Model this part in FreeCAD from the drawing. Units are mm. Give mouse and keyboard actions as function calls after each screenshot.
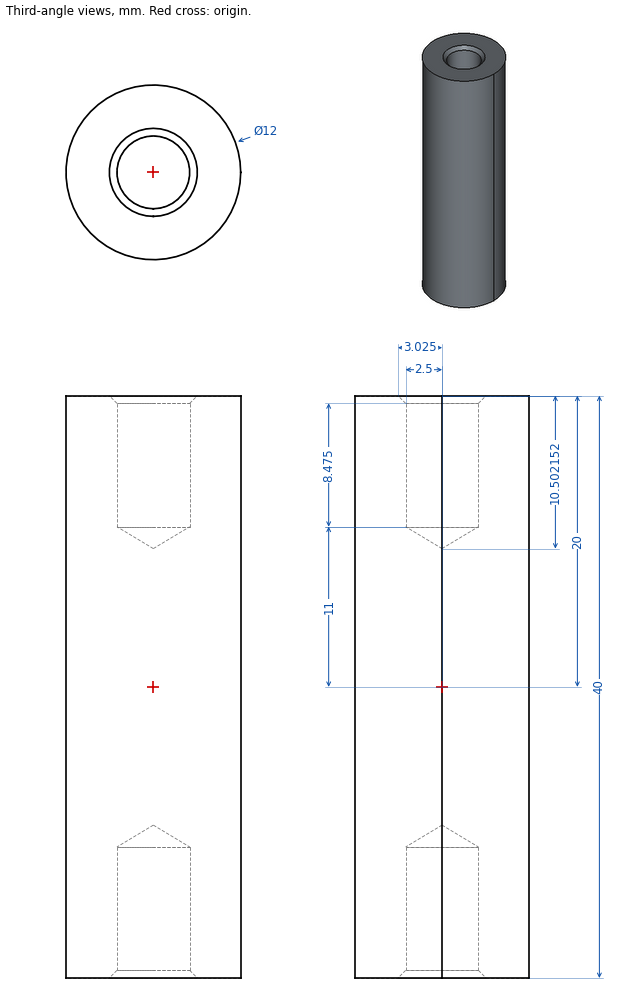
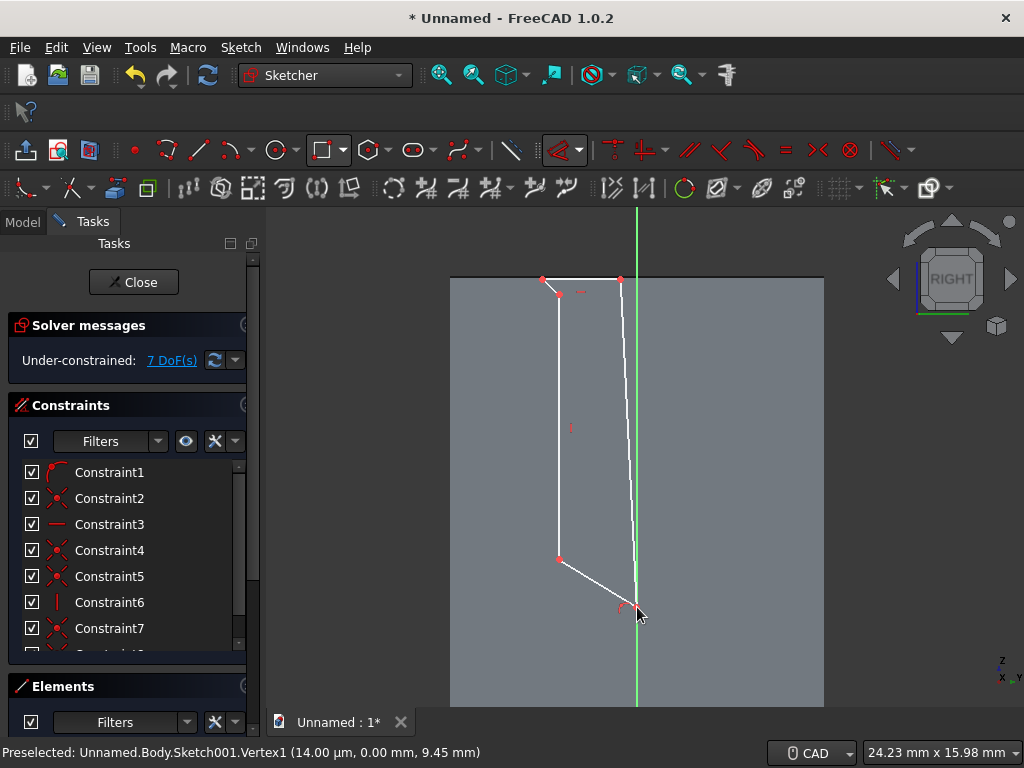
scroll(625, 378, up, 2)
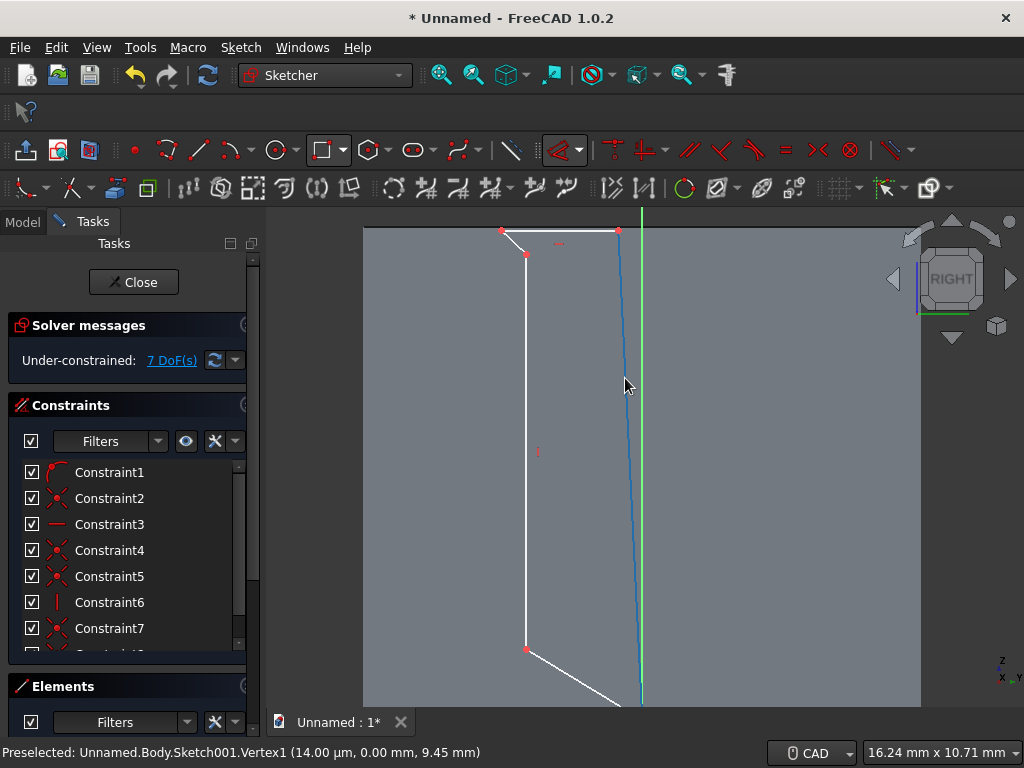
click(625, 377)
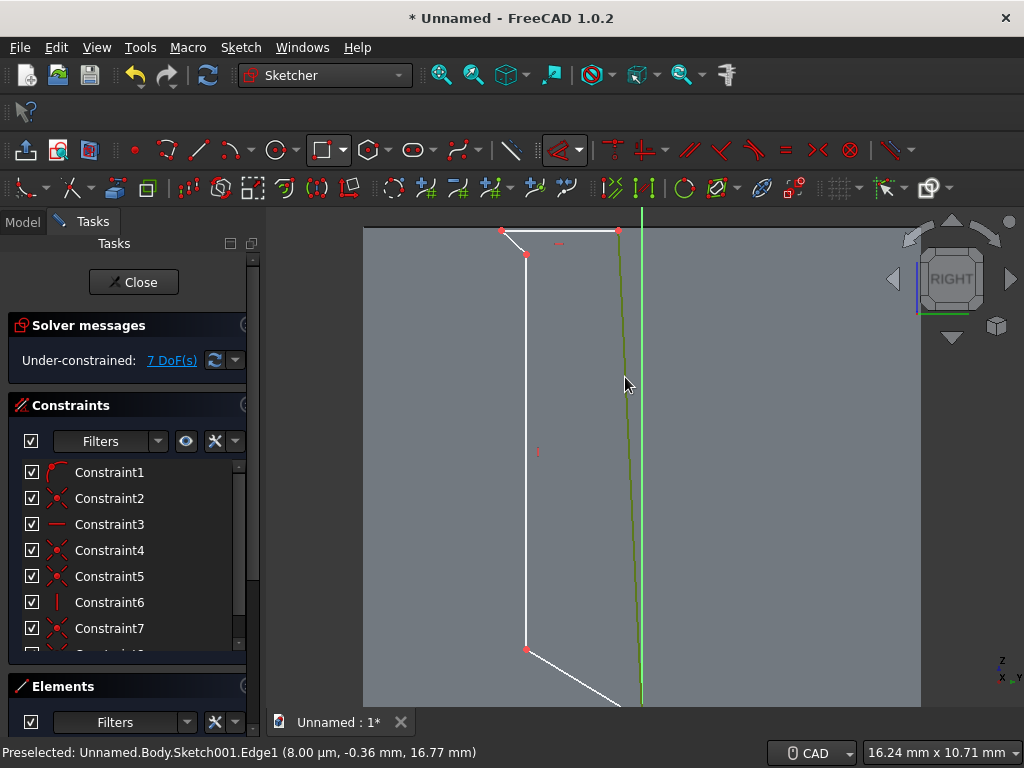
click(668, 150)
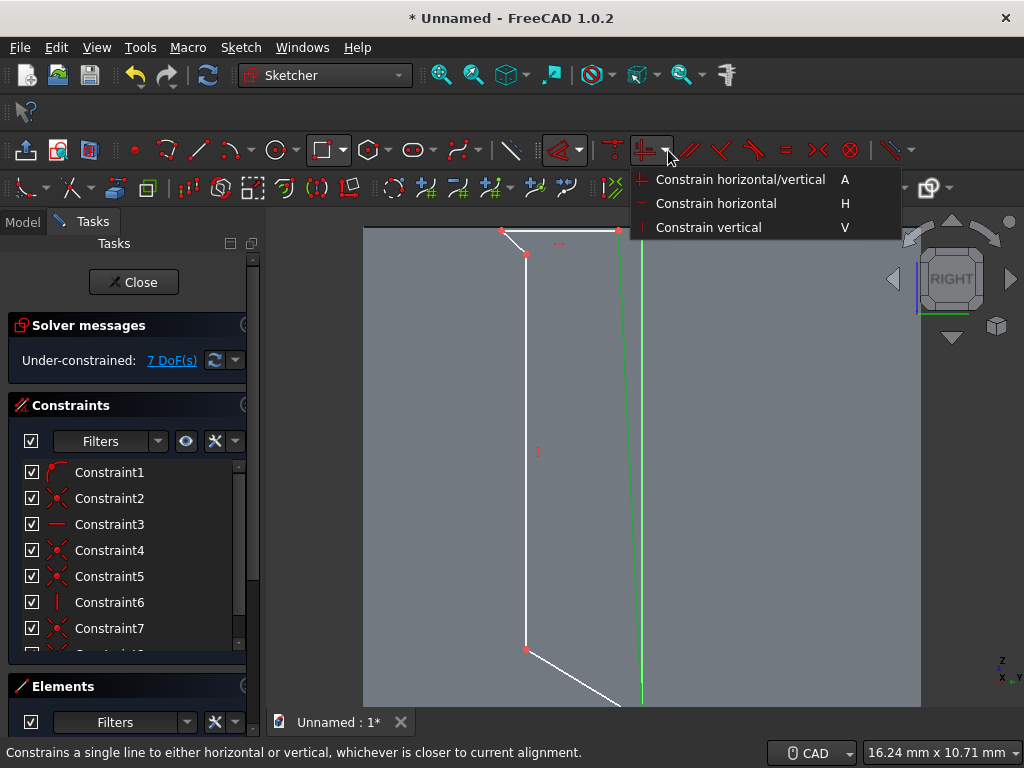
click(766, 227)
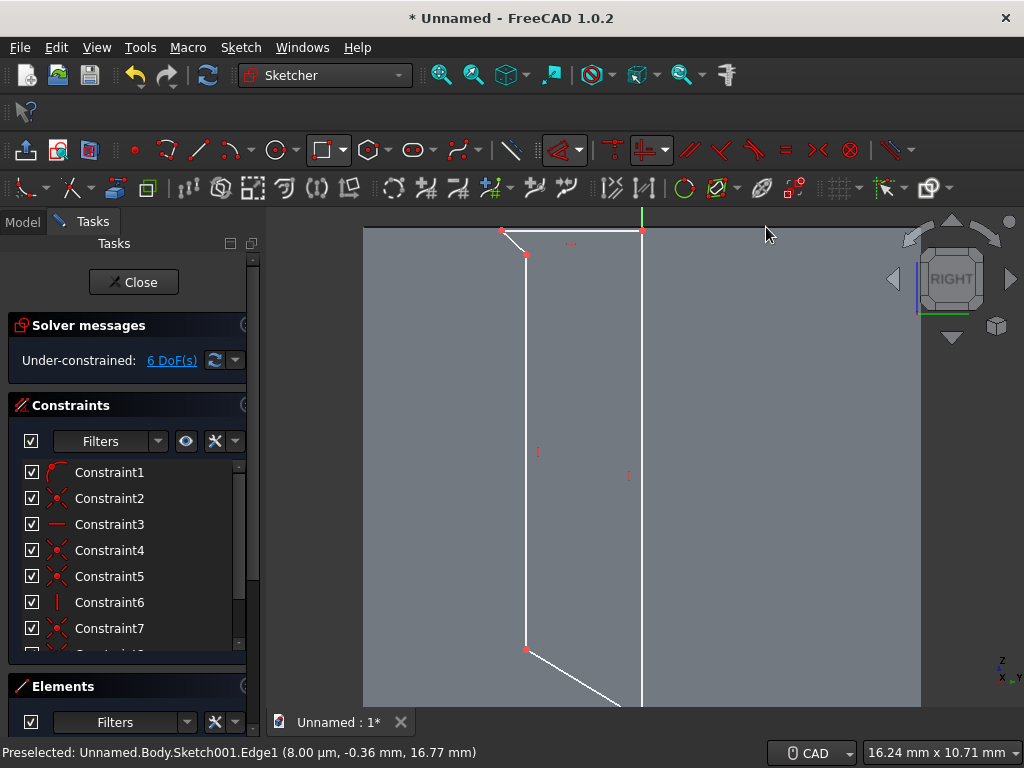
scroll(579, 319, down, 5)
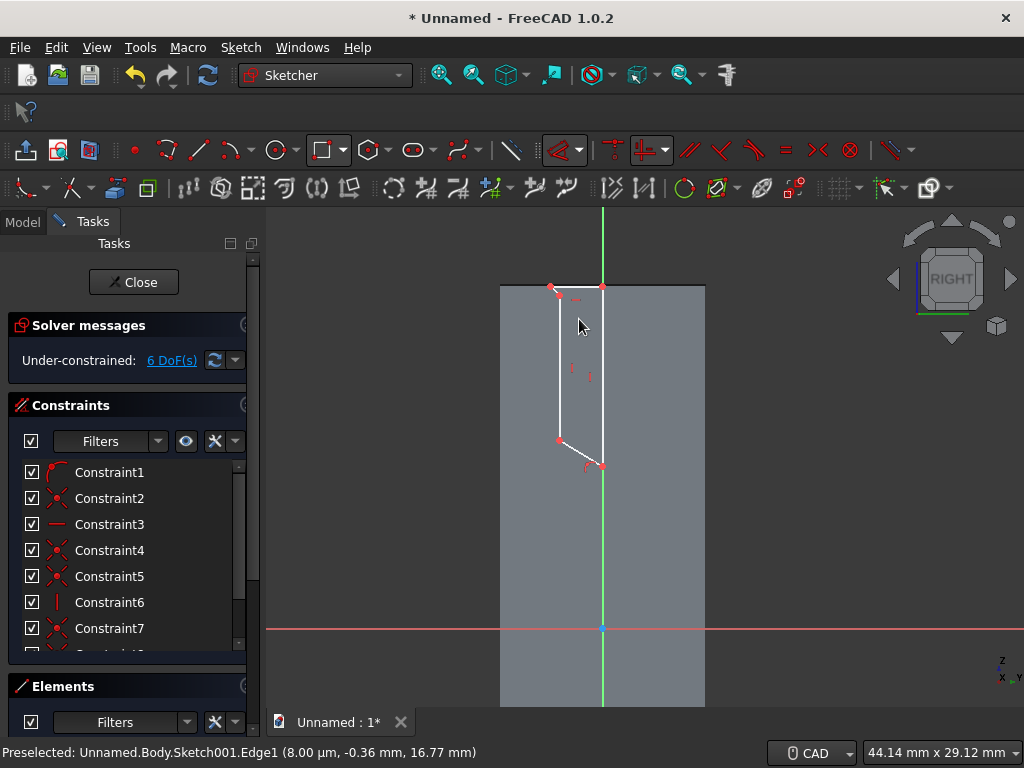
click(603, 287)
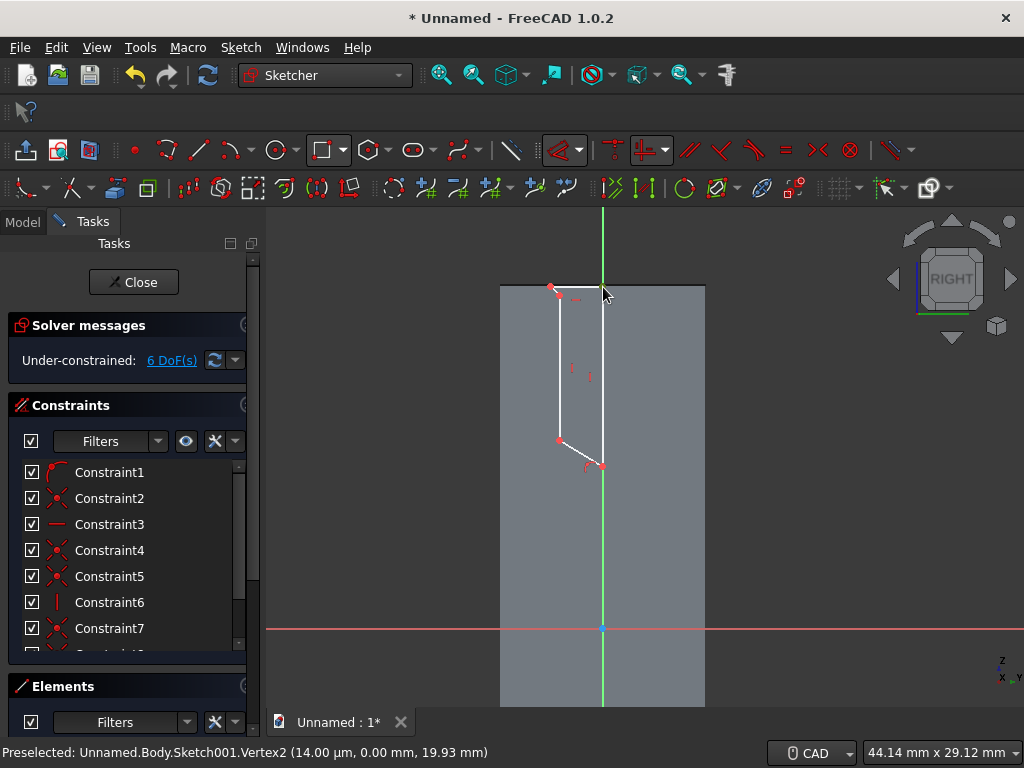
click(582, 150)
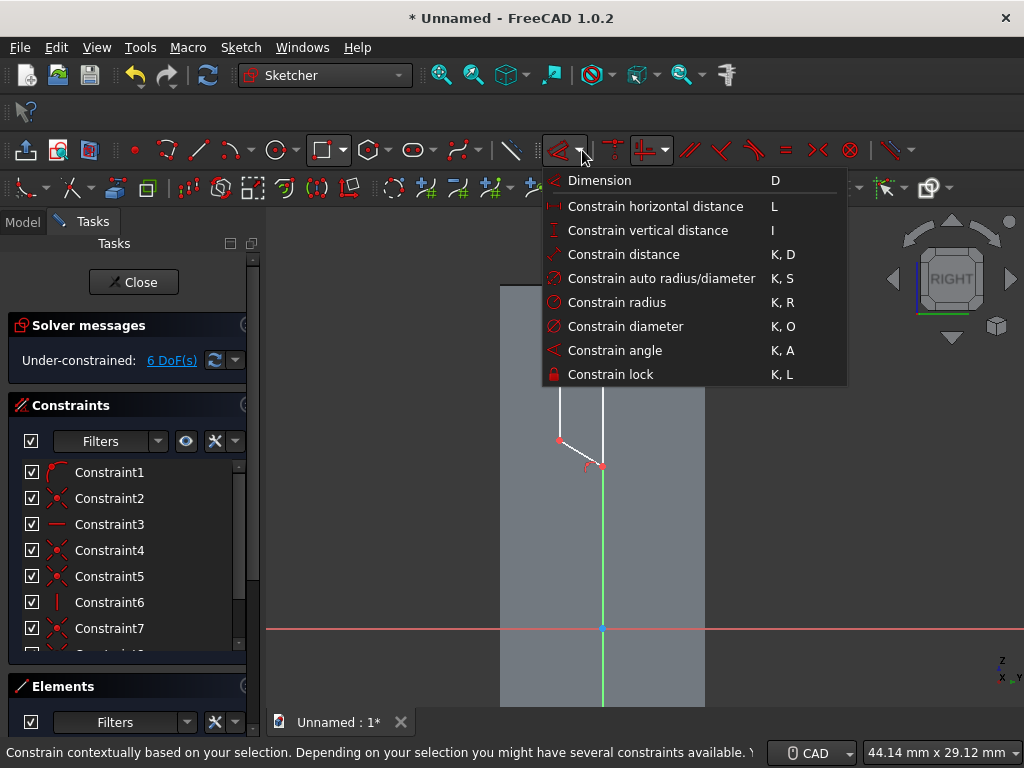
click(695, 230)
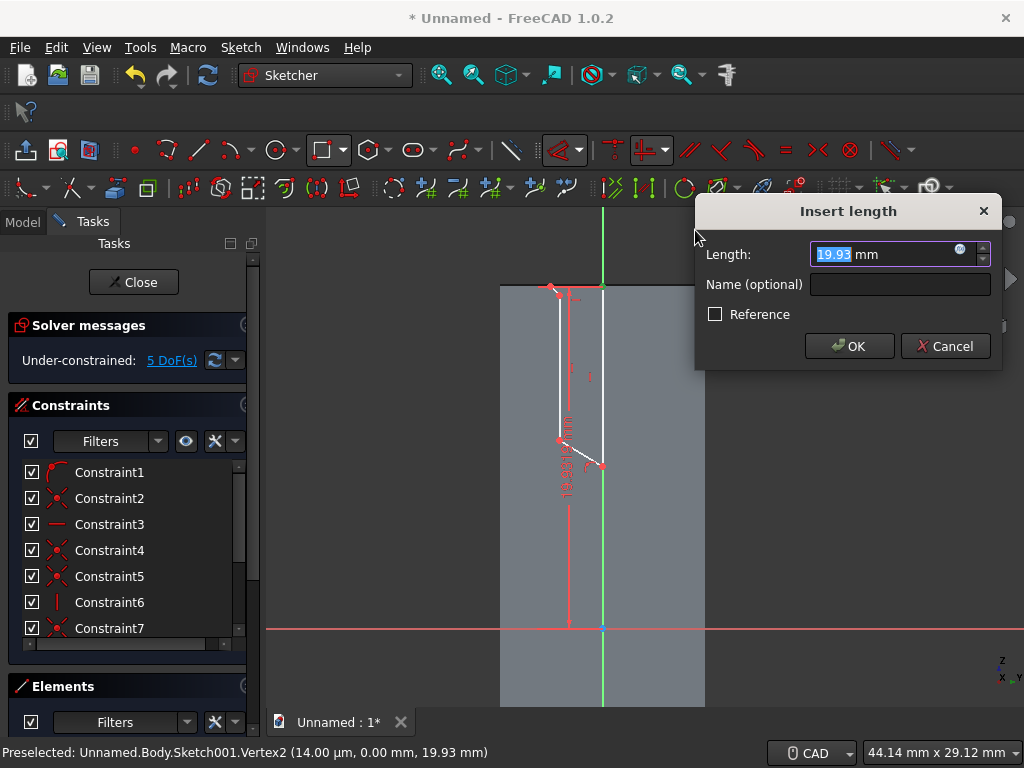
text(20)
key(Return)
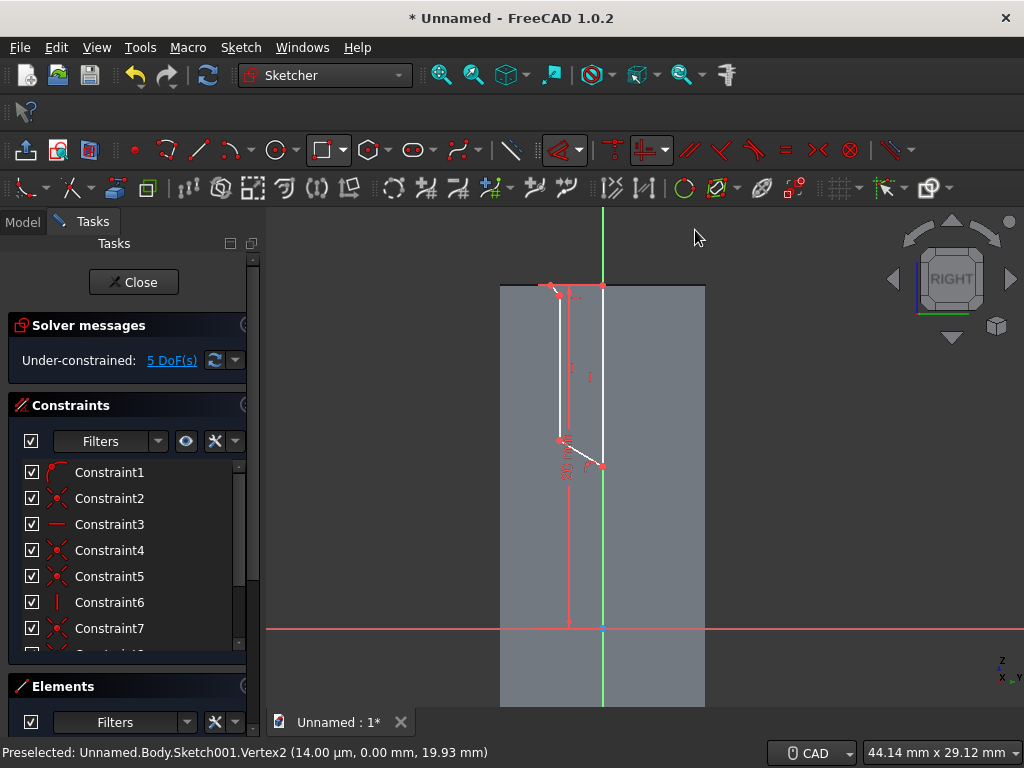
click(560, 441)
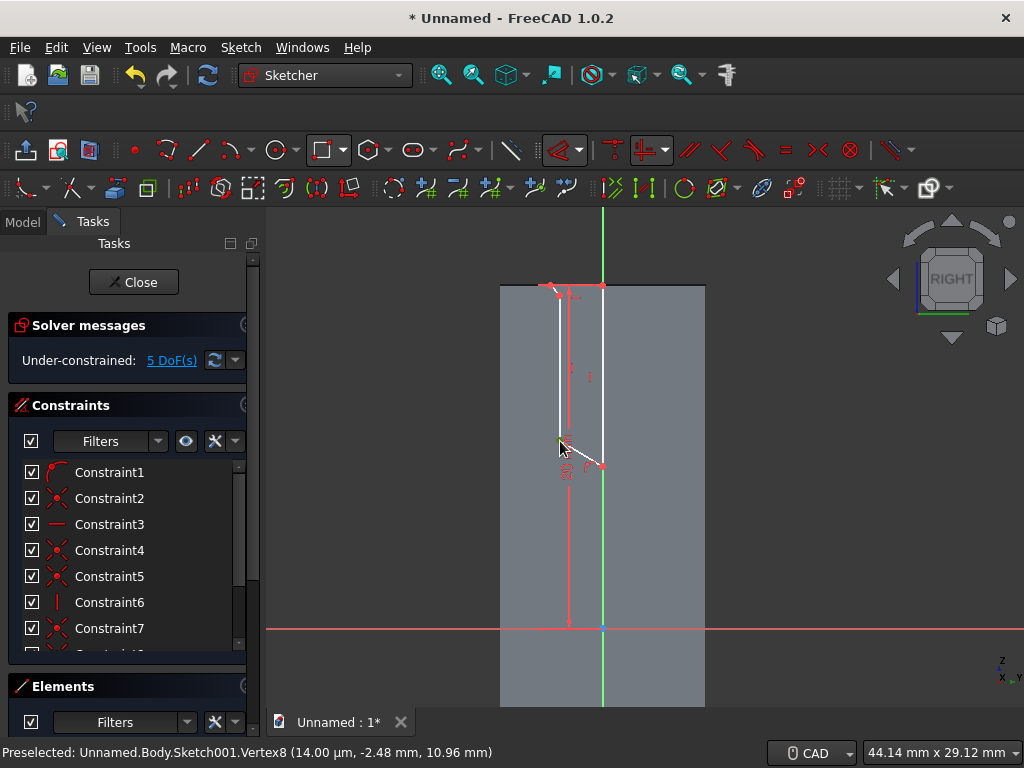
click(582, 150)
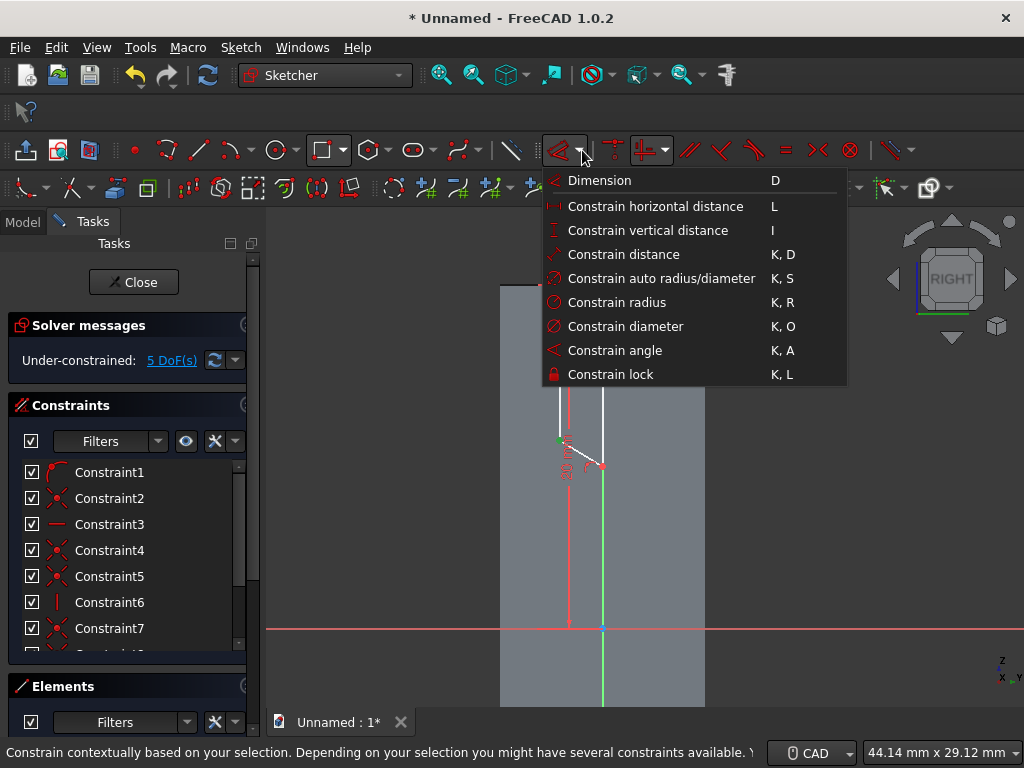
click(695, 230)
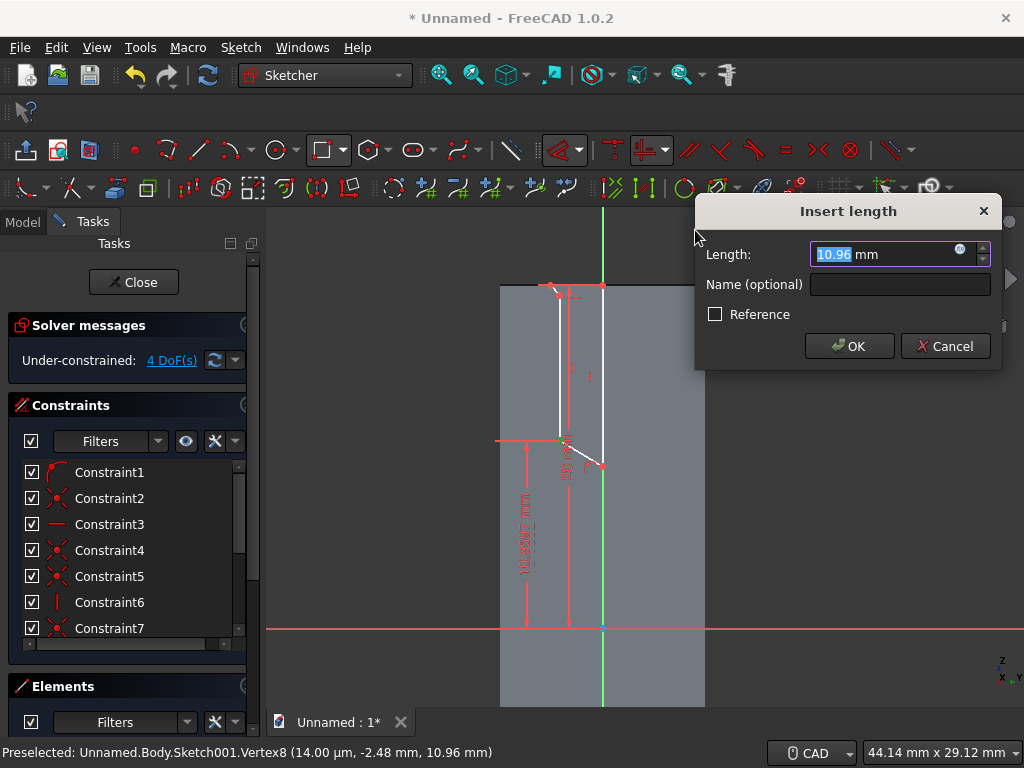
text(11)
key(Return)